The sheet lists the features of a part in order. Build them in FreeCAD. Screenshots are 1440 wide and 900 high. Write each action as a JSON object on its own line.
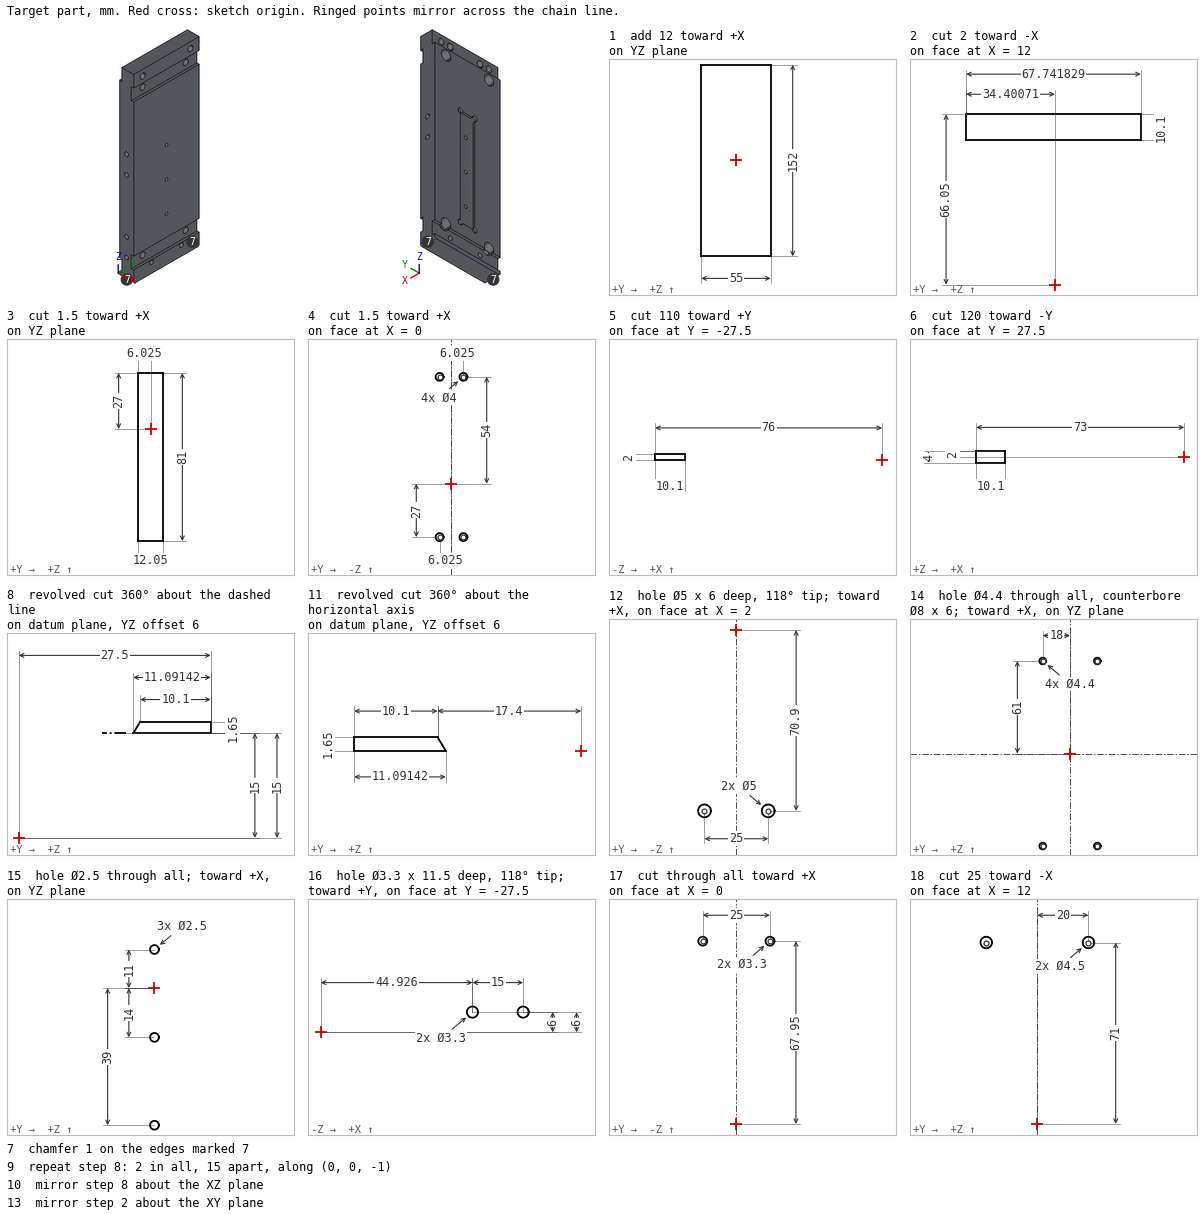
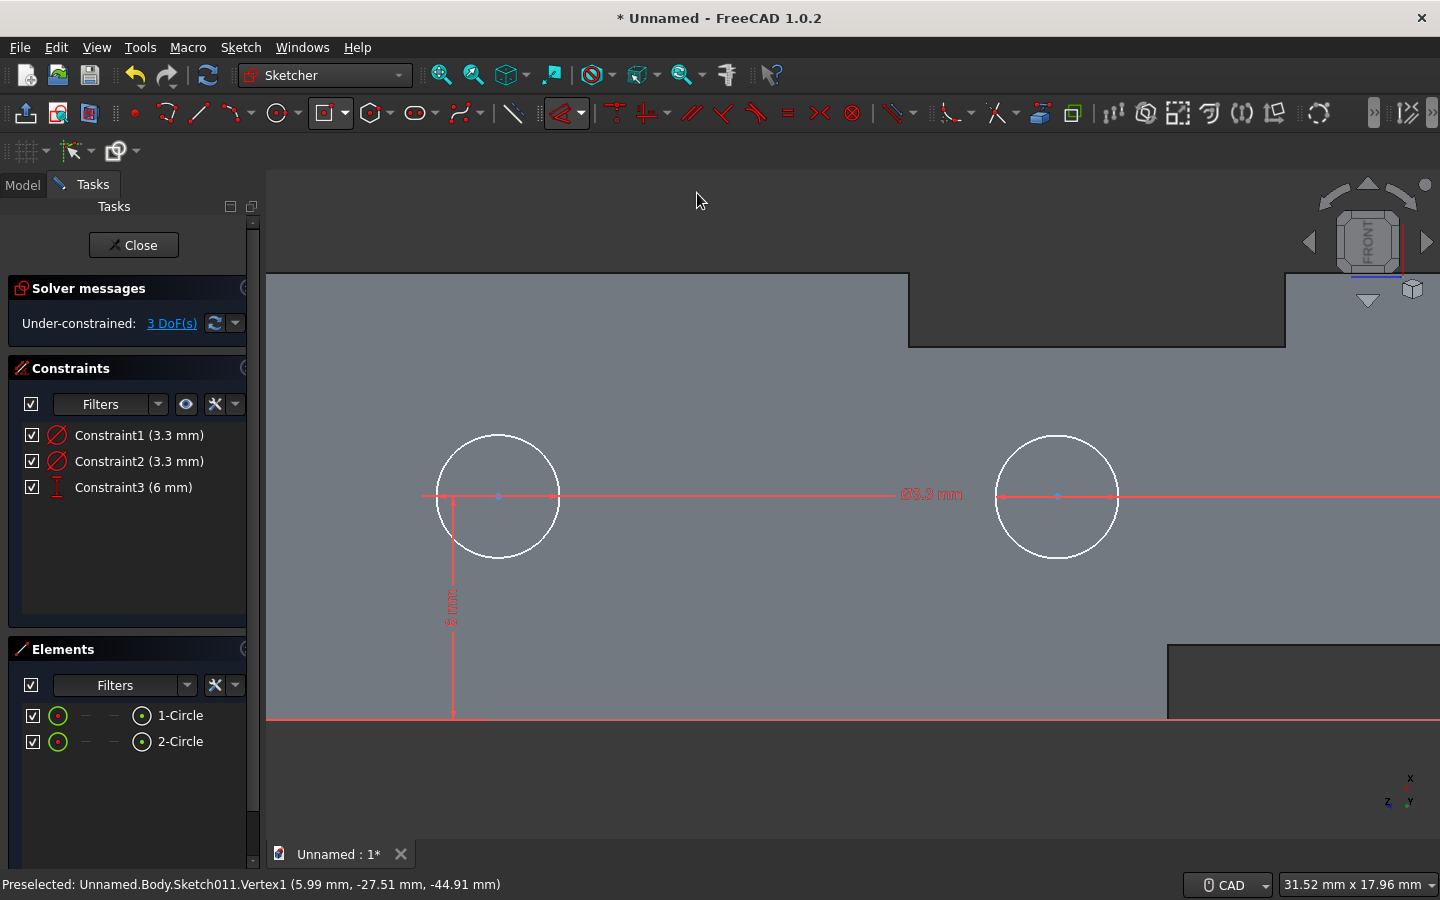
{"action": "left_click", "coordinate": [1057, 497]}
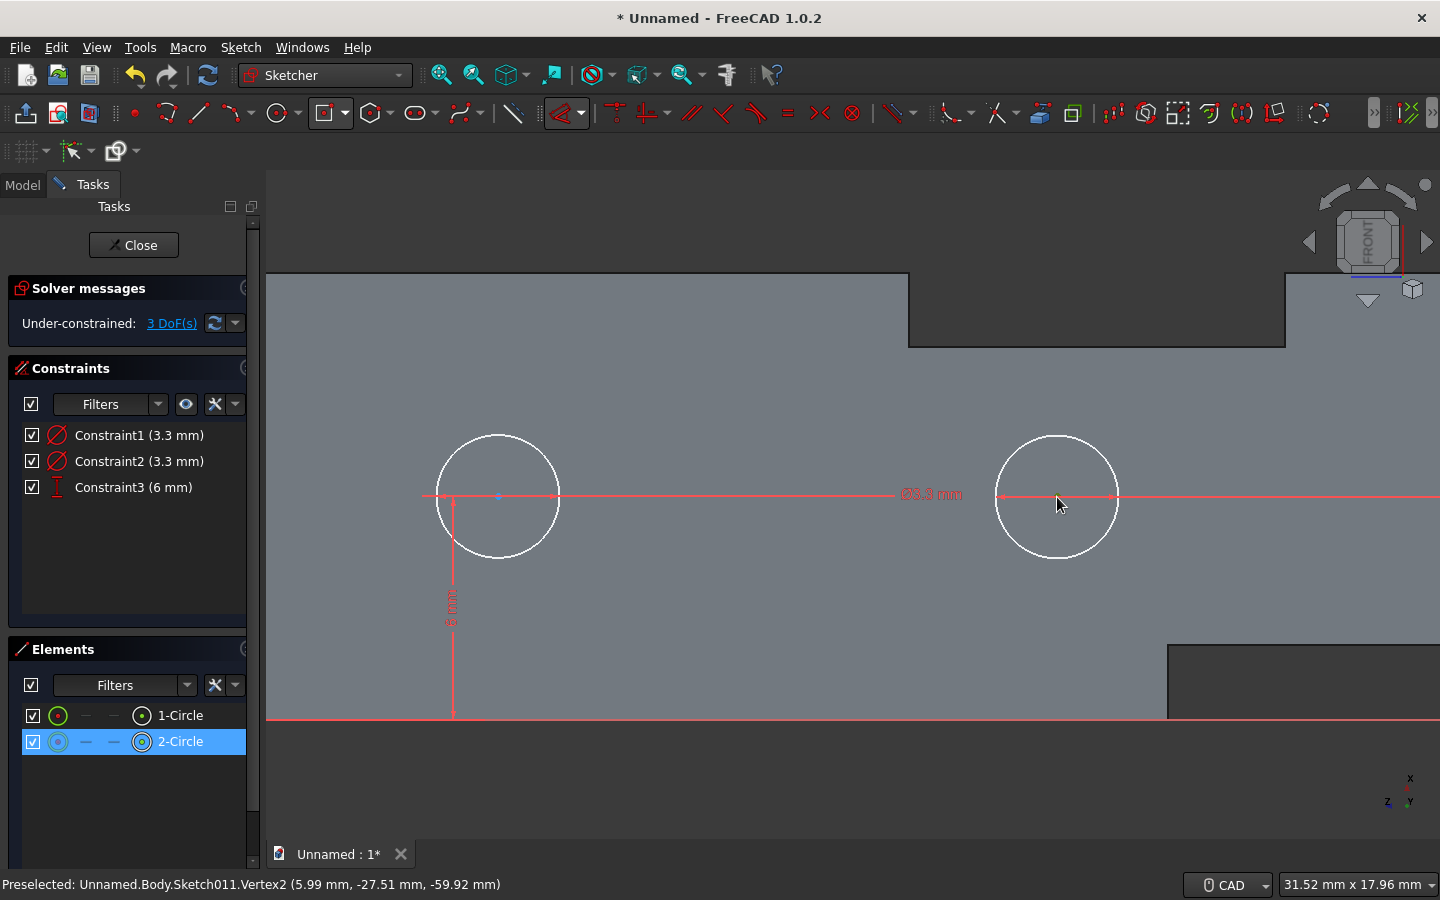
{"action": "left_click", "coordinate": [584, 114]}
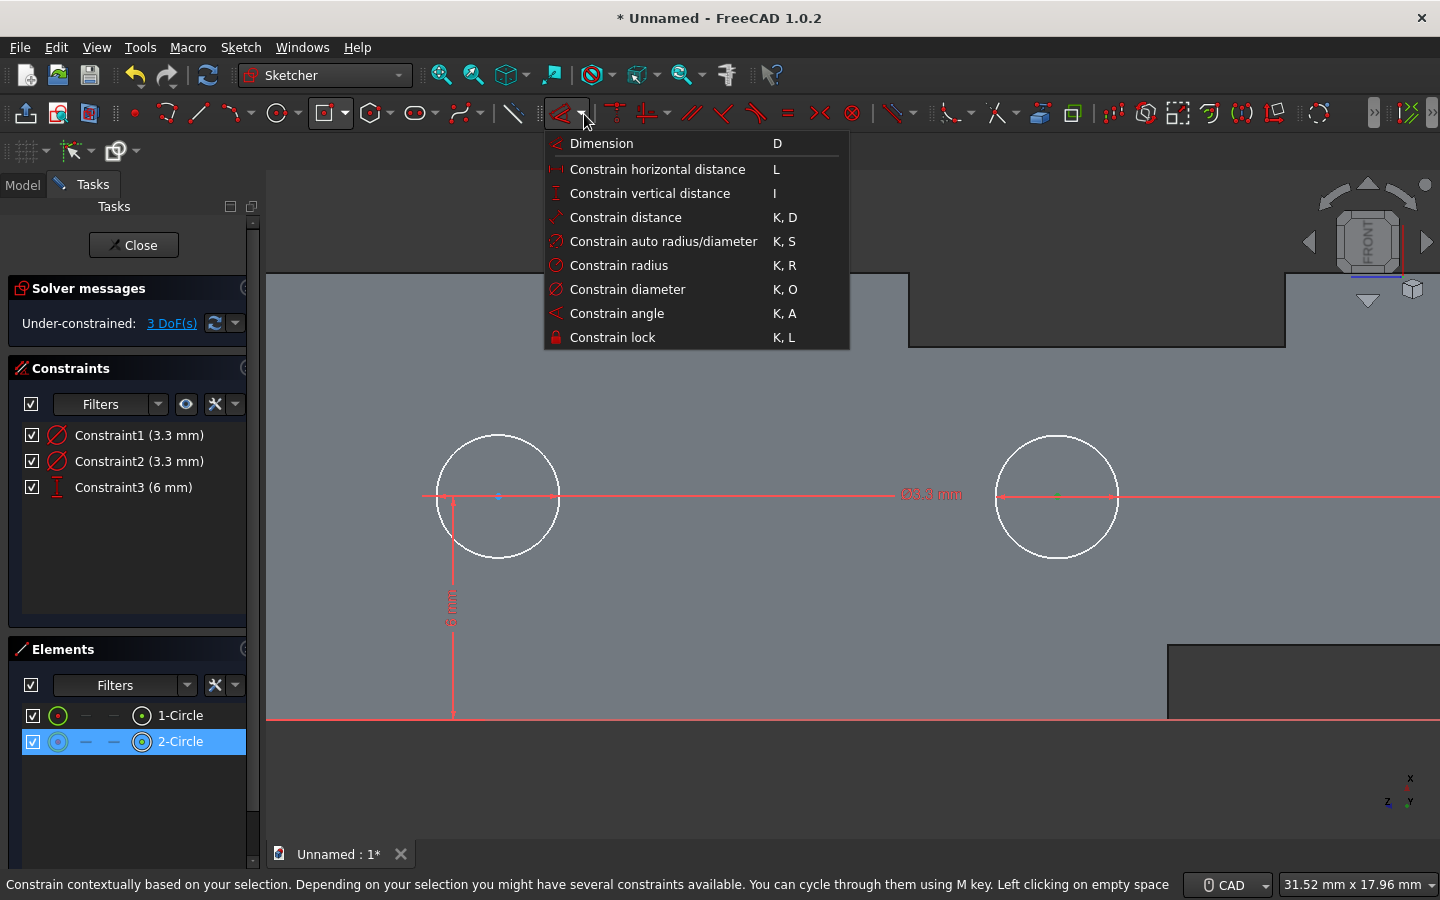
{"action": "left_click", "coordinate": [697, 193]}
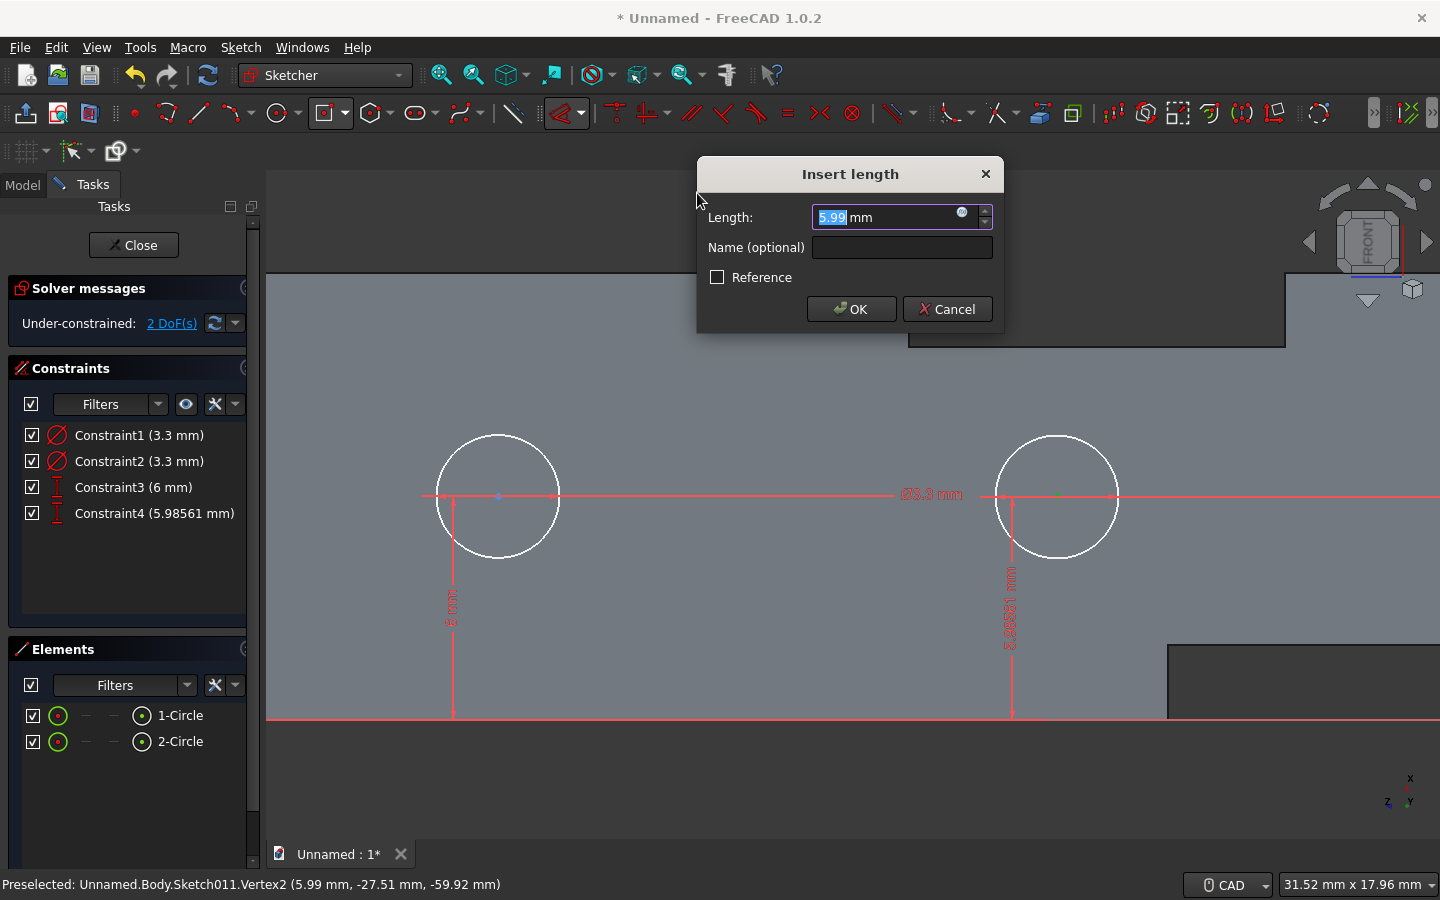
{"action": "type", "text": "6"}
{"action": "key", "text": "Return"}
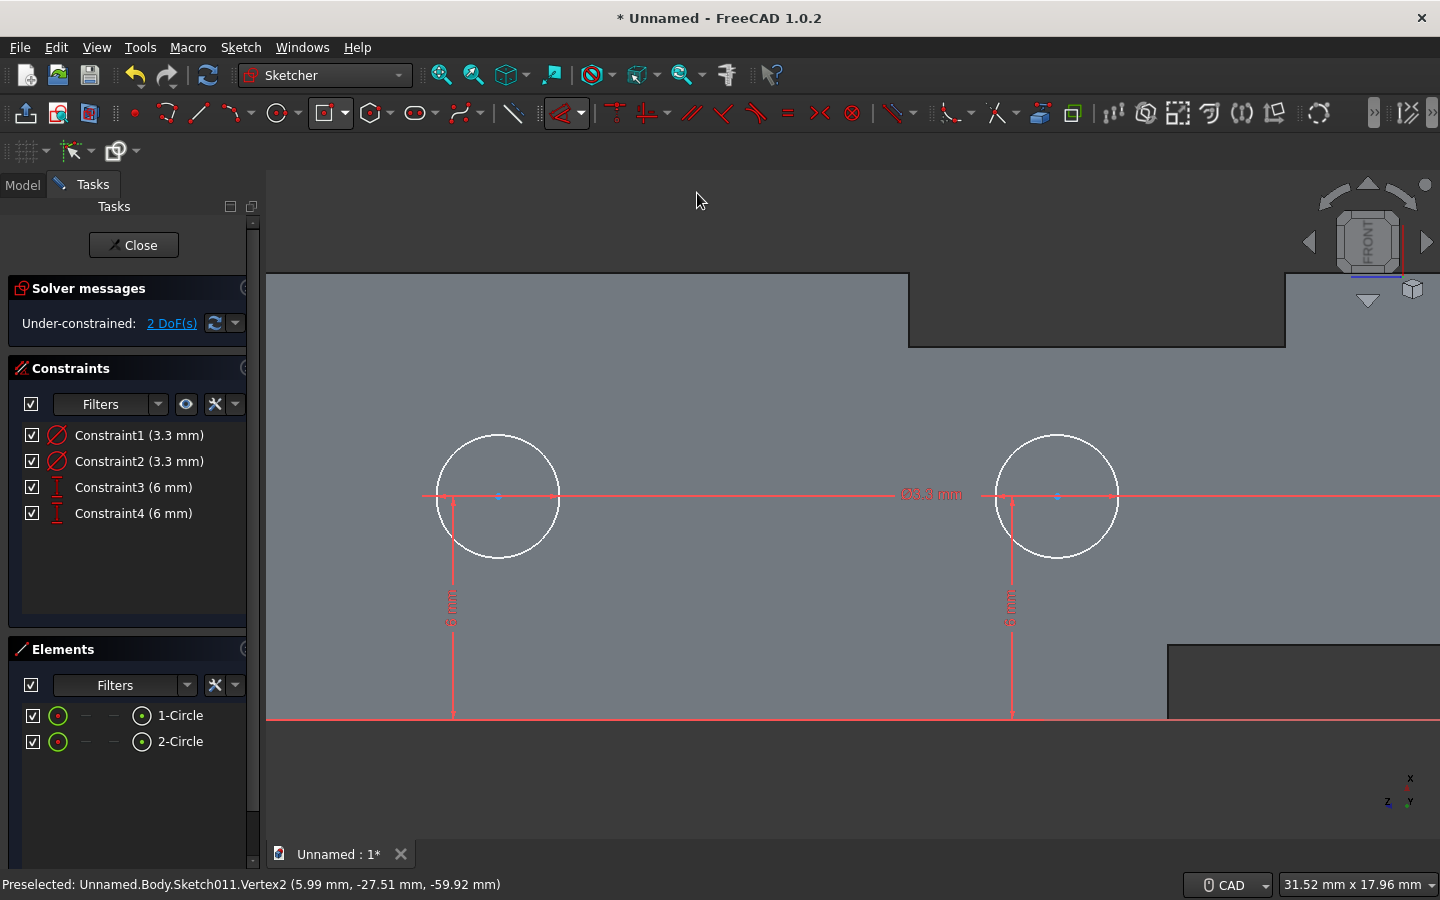
{"action": "left_click", "coordinate": [498, 496]}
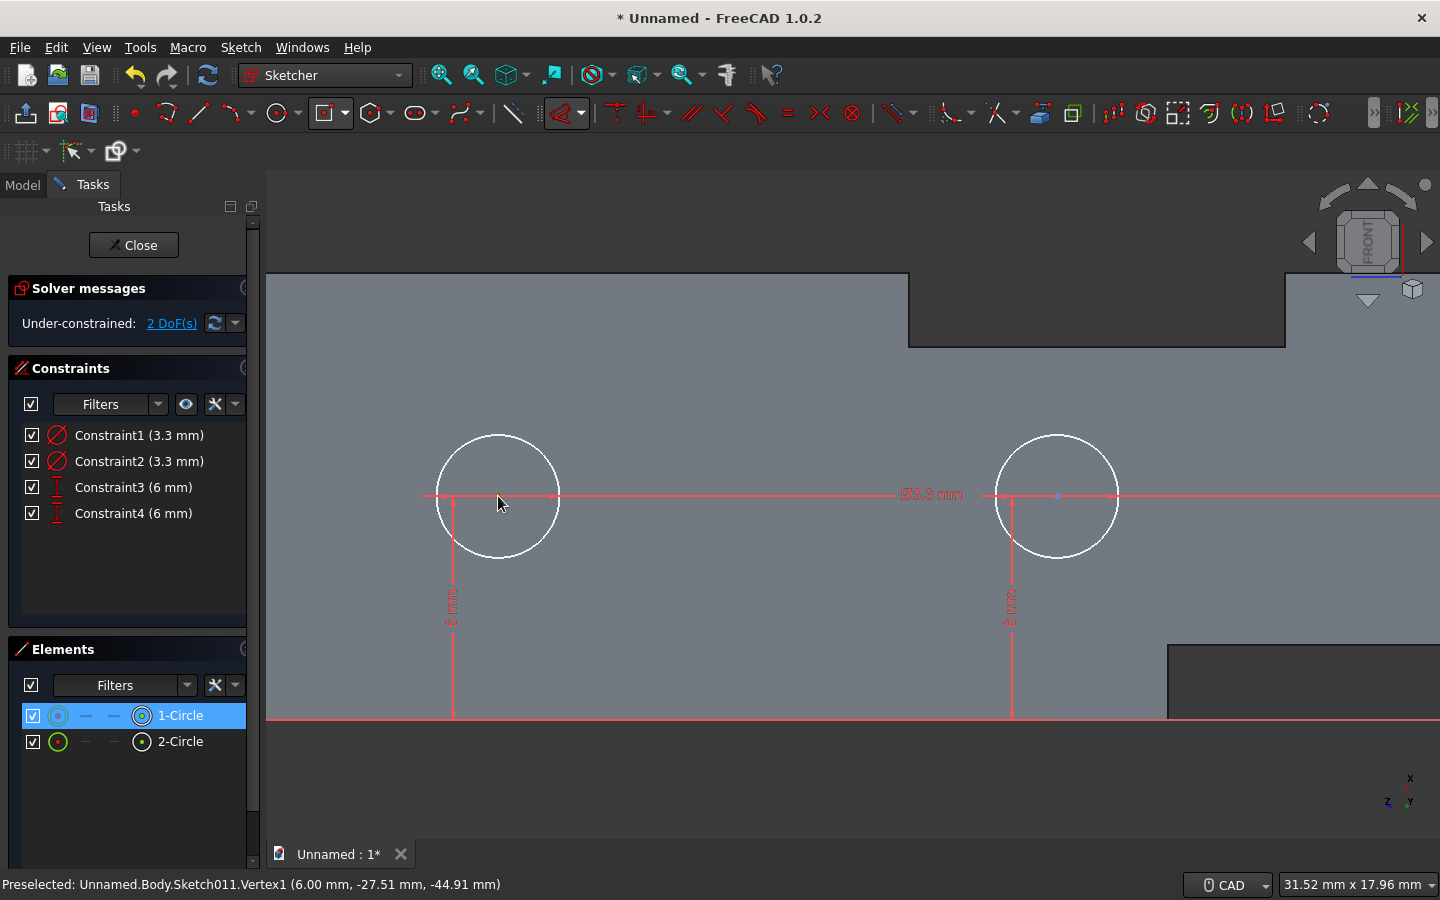
{"action": "left_click", "coordinate": [1057, 496]}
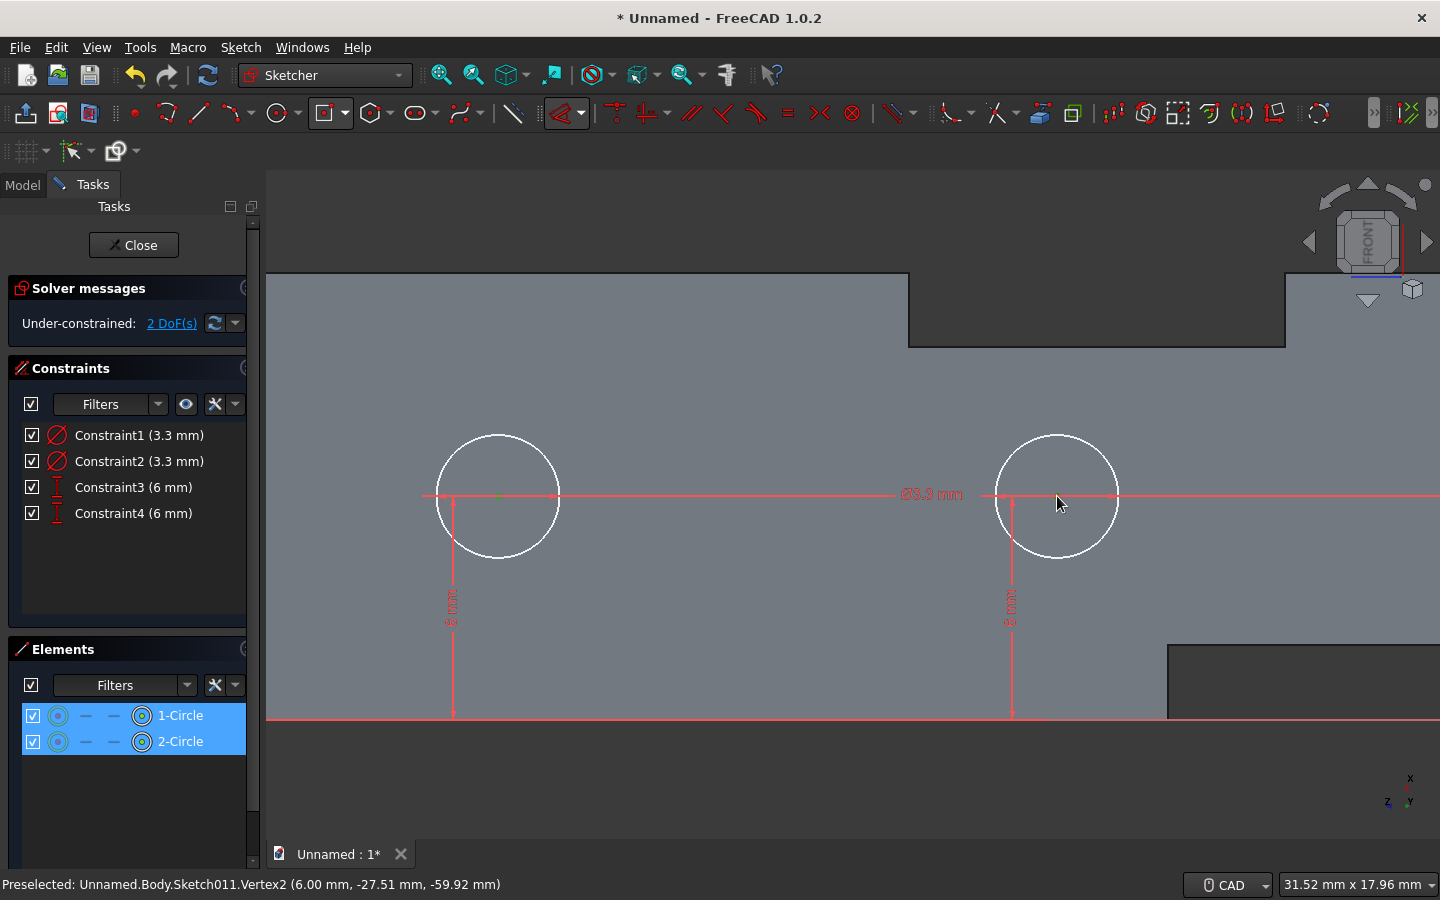
{"action": "key", "text": "l"}